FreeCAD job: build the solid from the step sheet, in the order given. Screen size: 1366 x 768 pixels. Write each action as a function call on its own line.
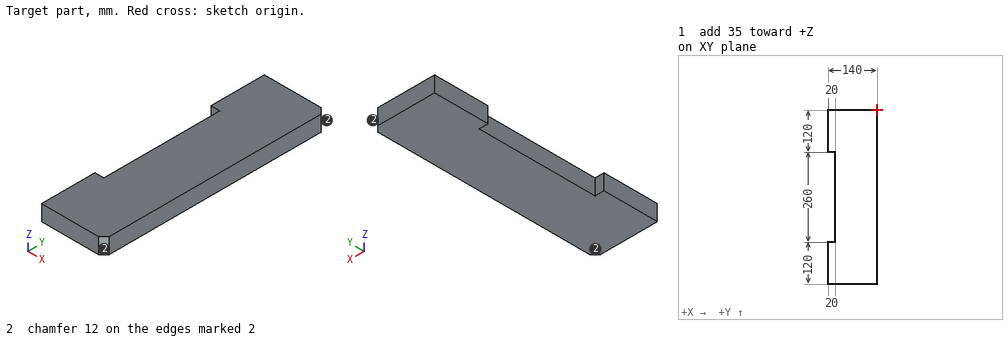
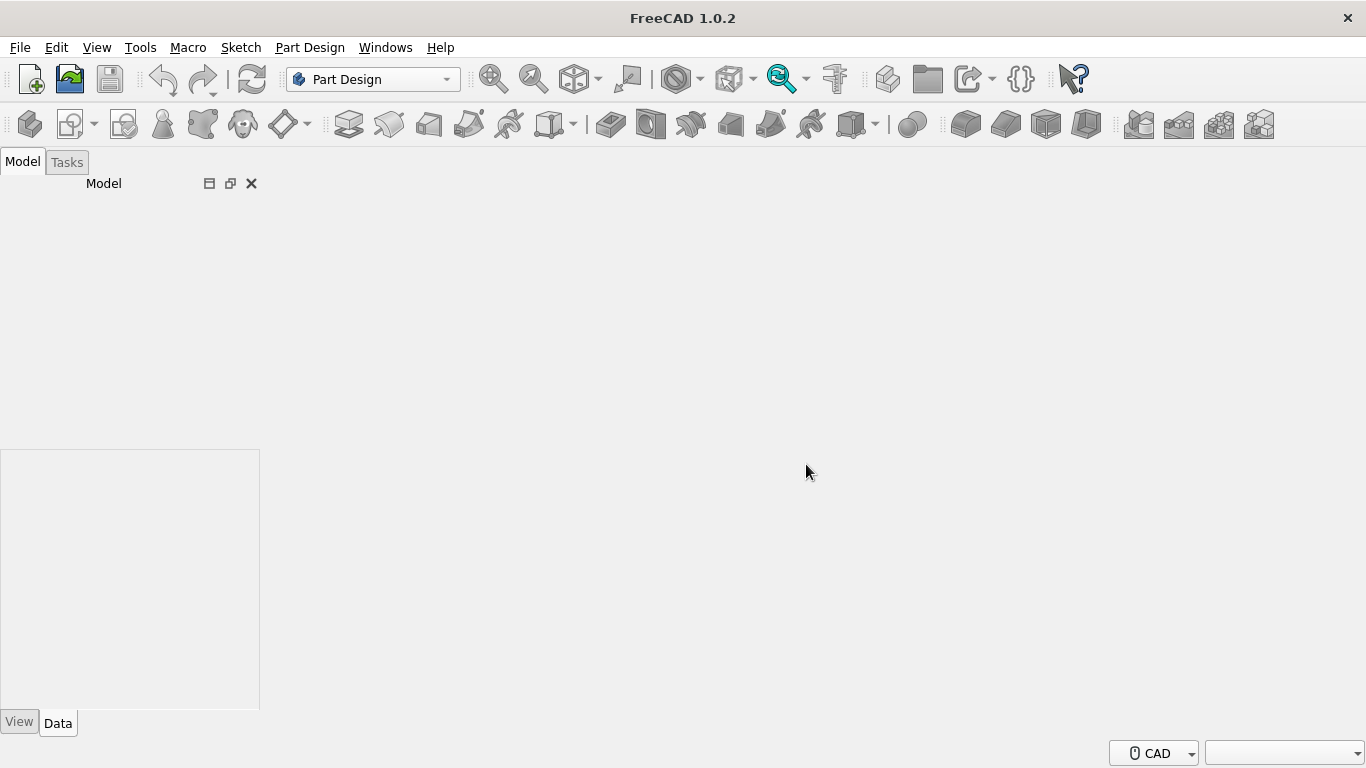
key(ctrl+n)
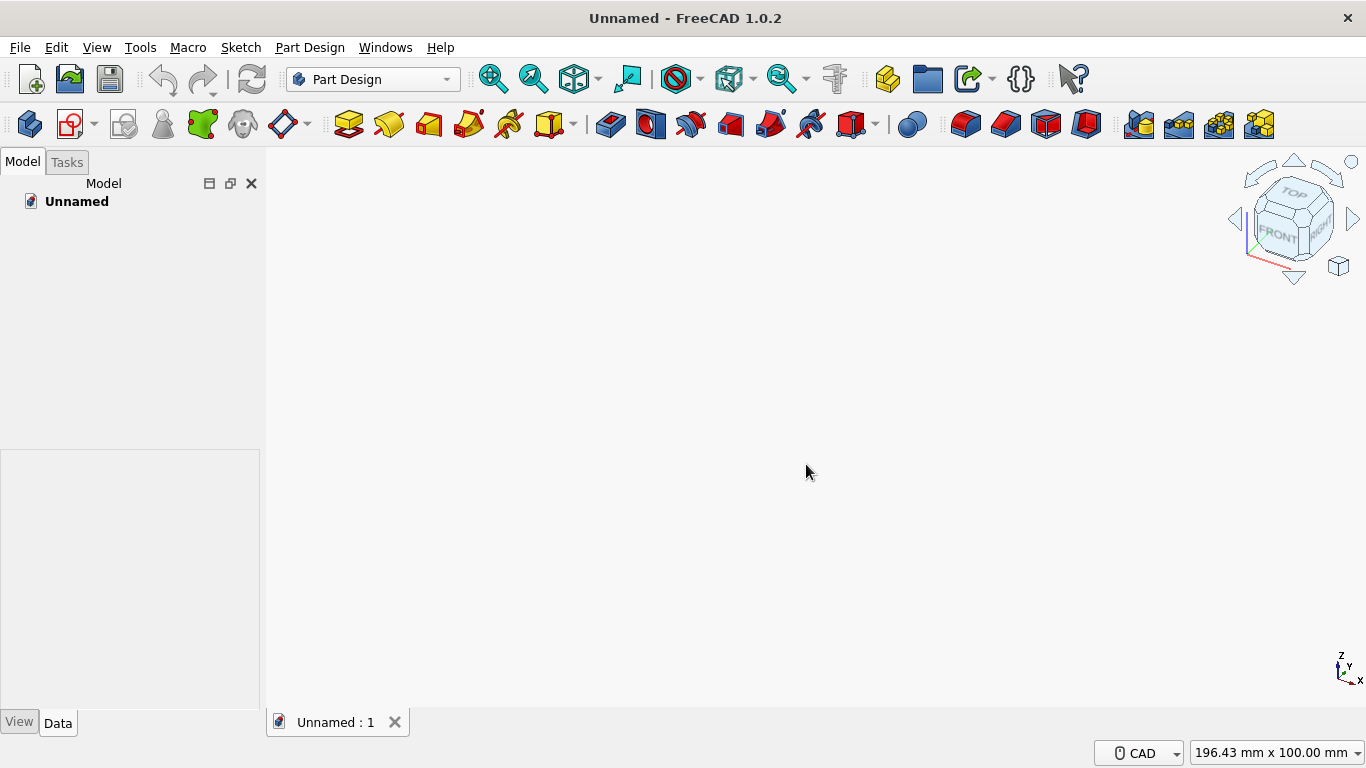
click(70, 124)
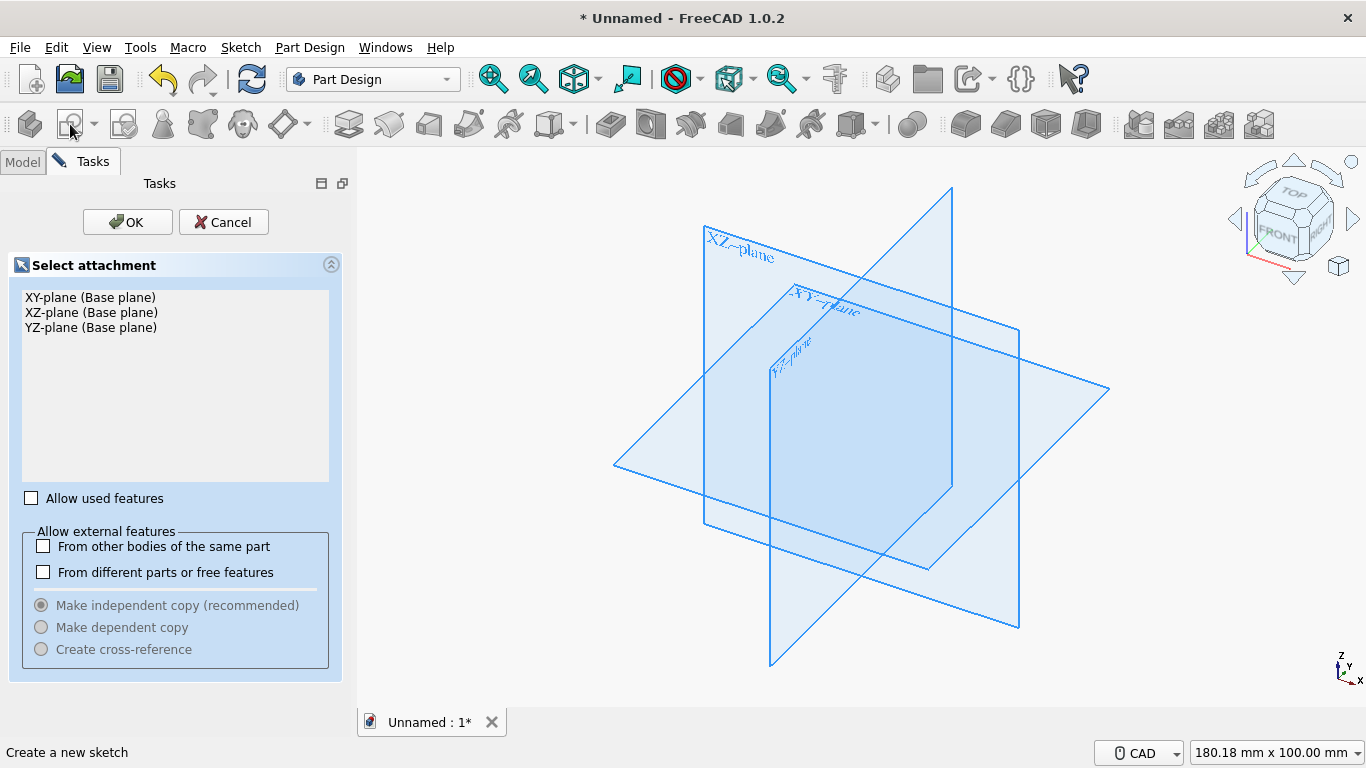
click(82, 298)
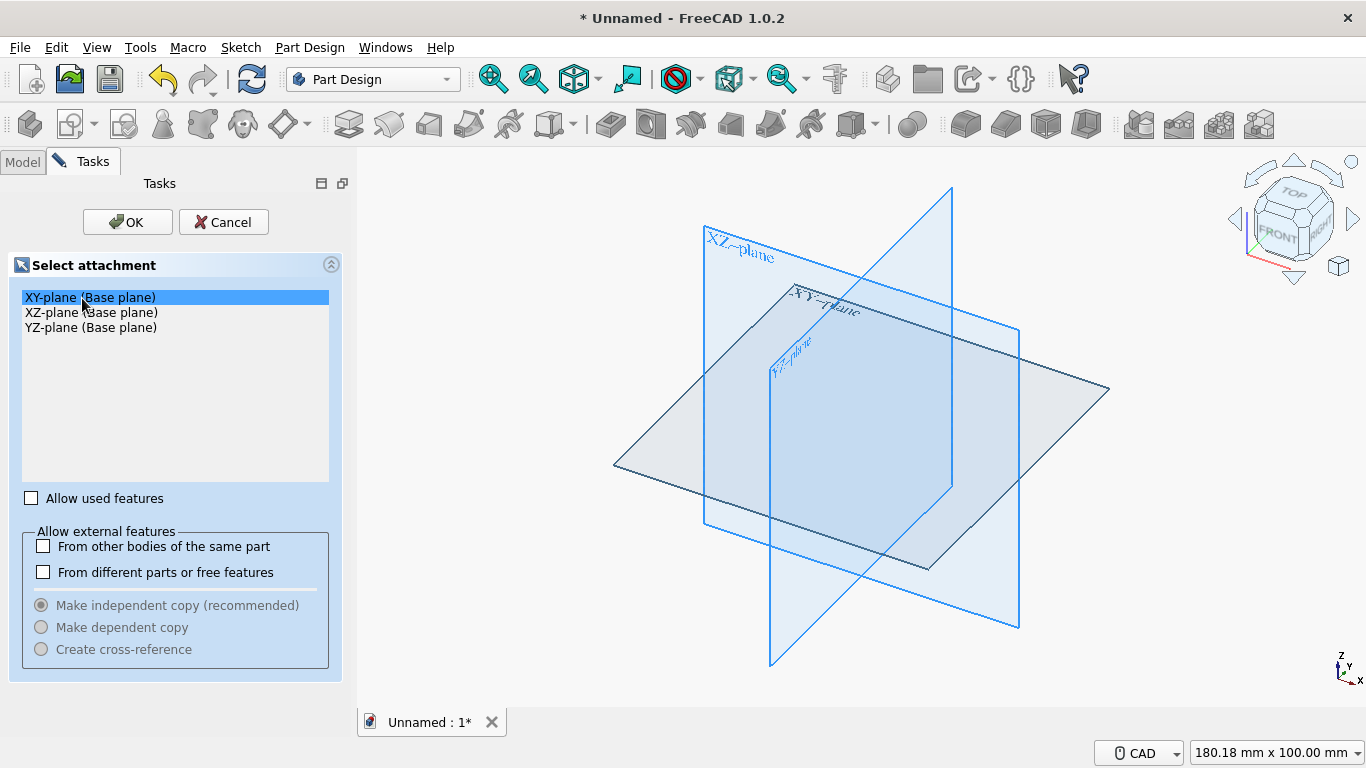
click(128, 222)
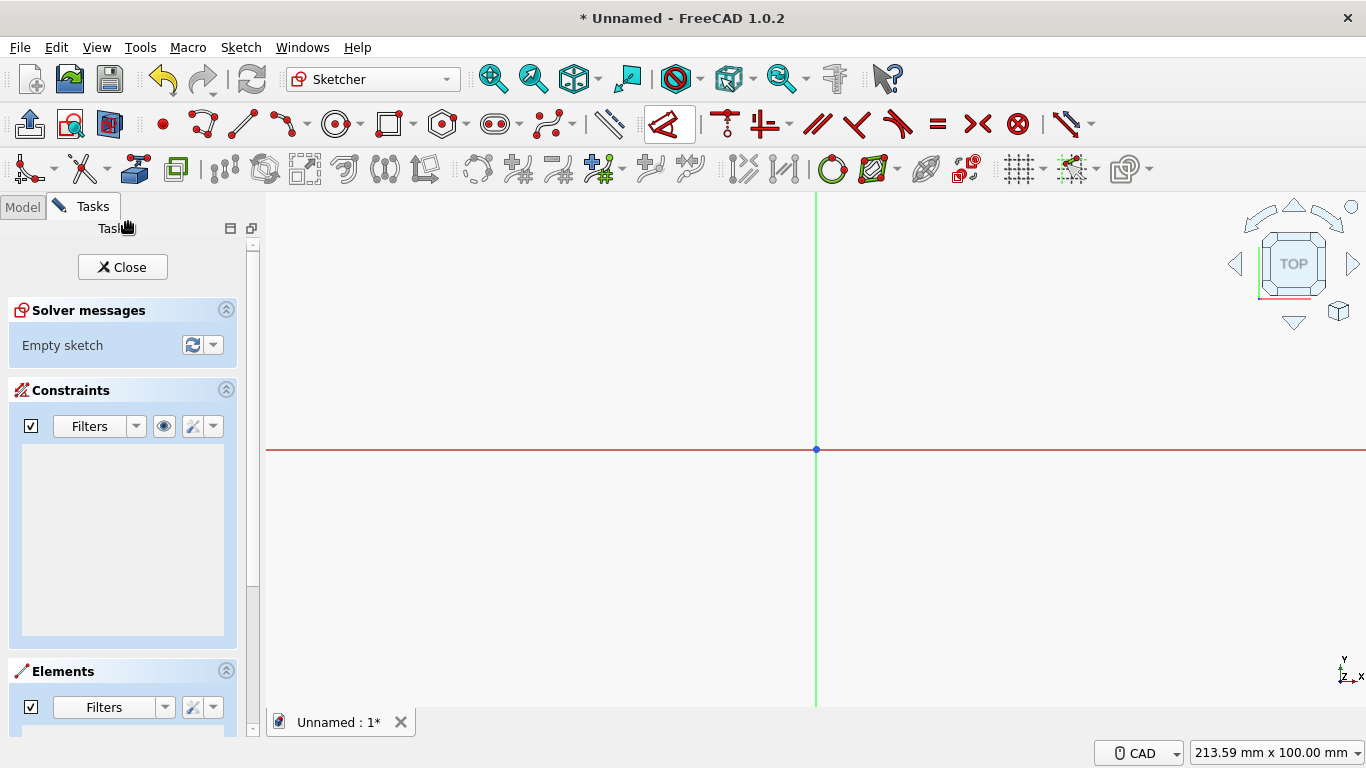
scroll(793, 248, down, 10)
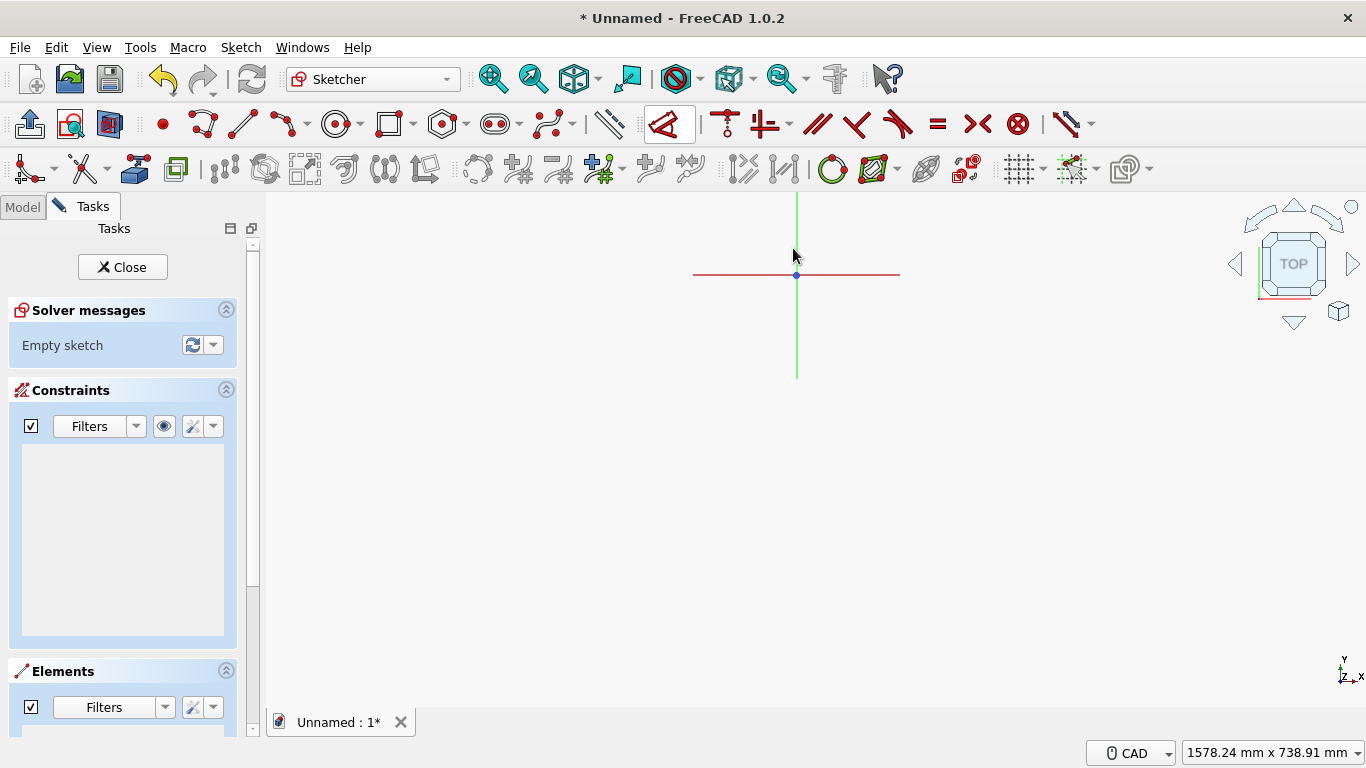
key(g)
key(m)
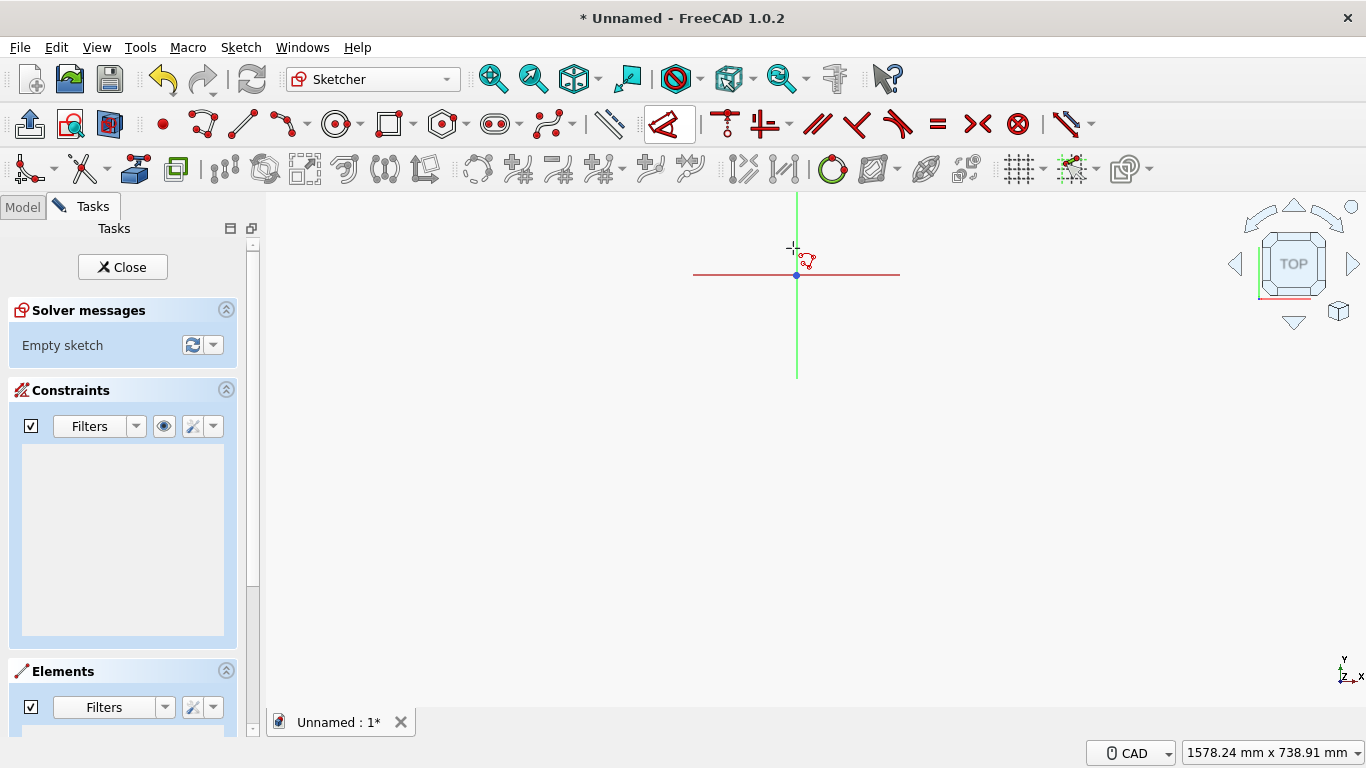
click(797, 275)
click(699, 284)
click(699, 359)
click(713, 359)
click(713, 540)
click(699, 540)
click(699, 624)
click(788, 624)
click(797, 275)
key(Escape)
key(Escape)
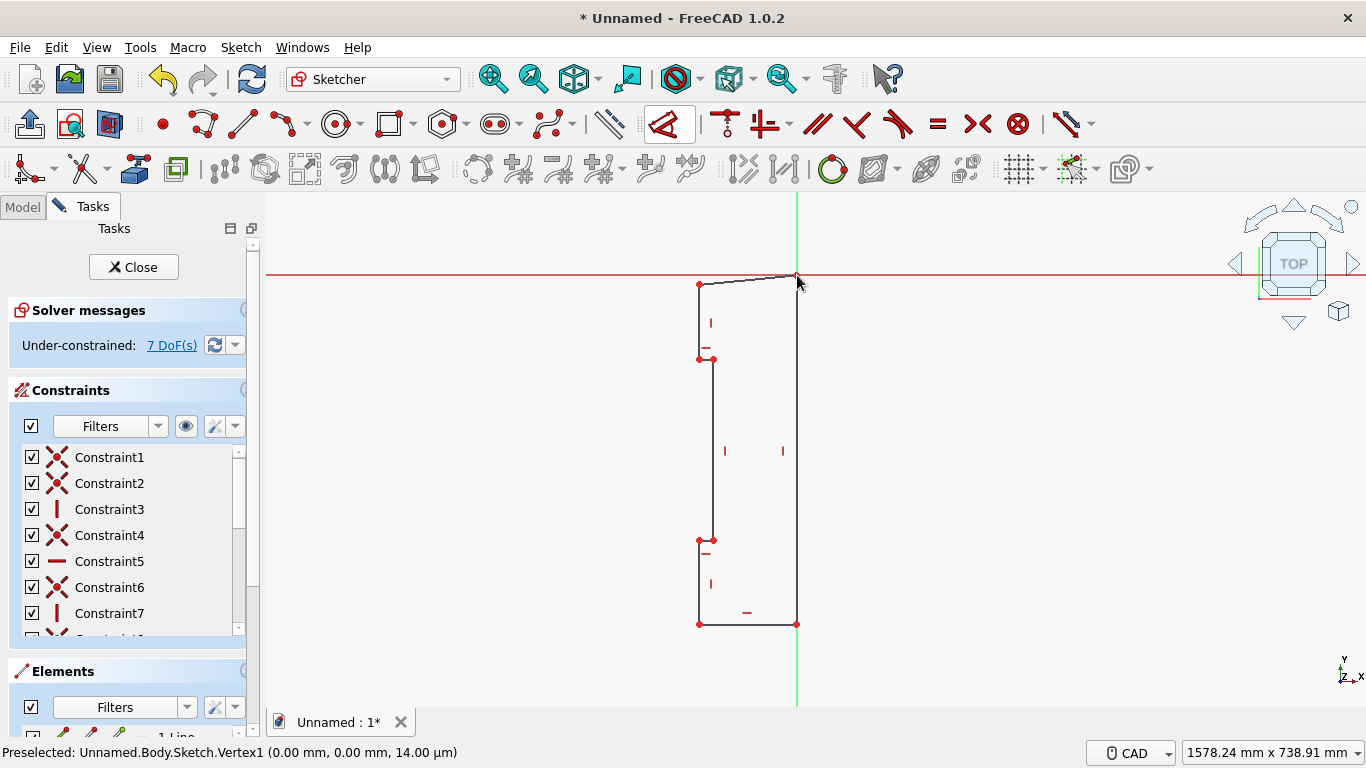
click(767, 278)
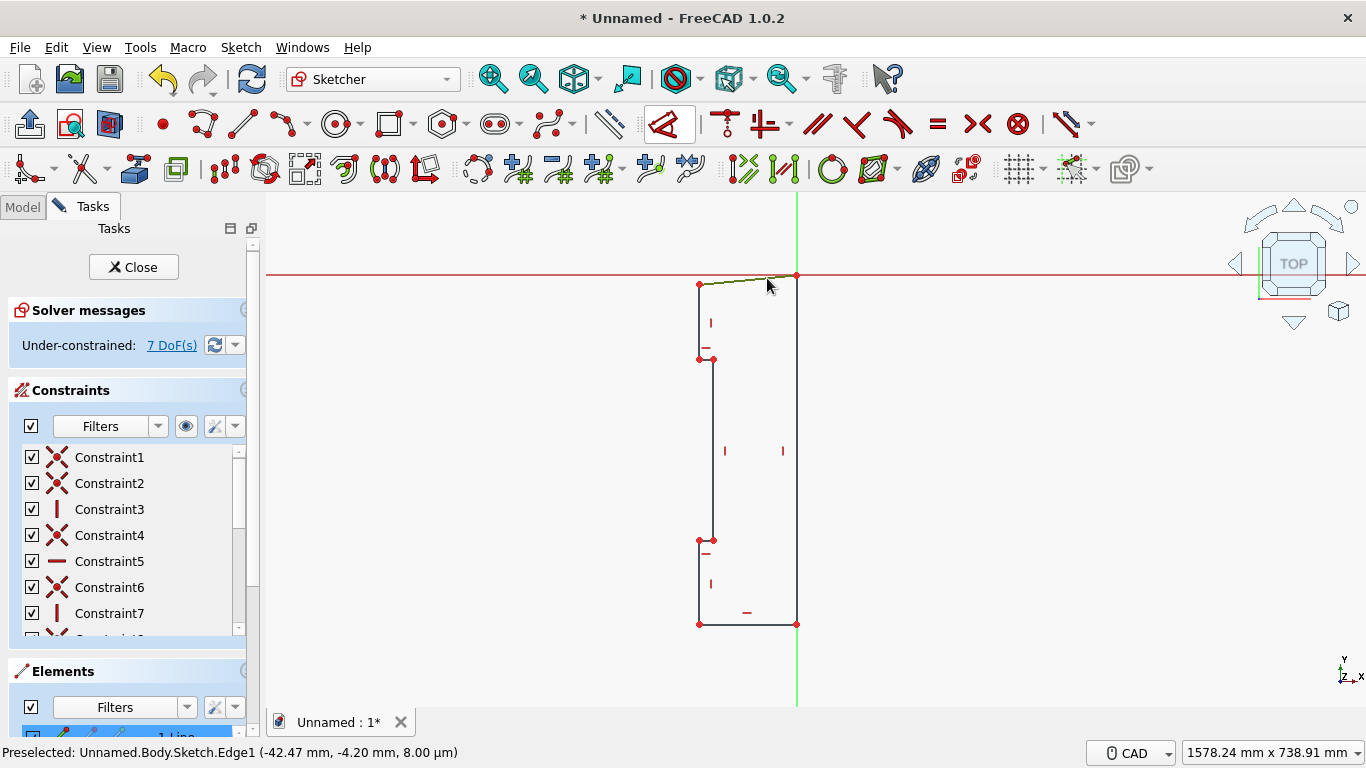
key(h)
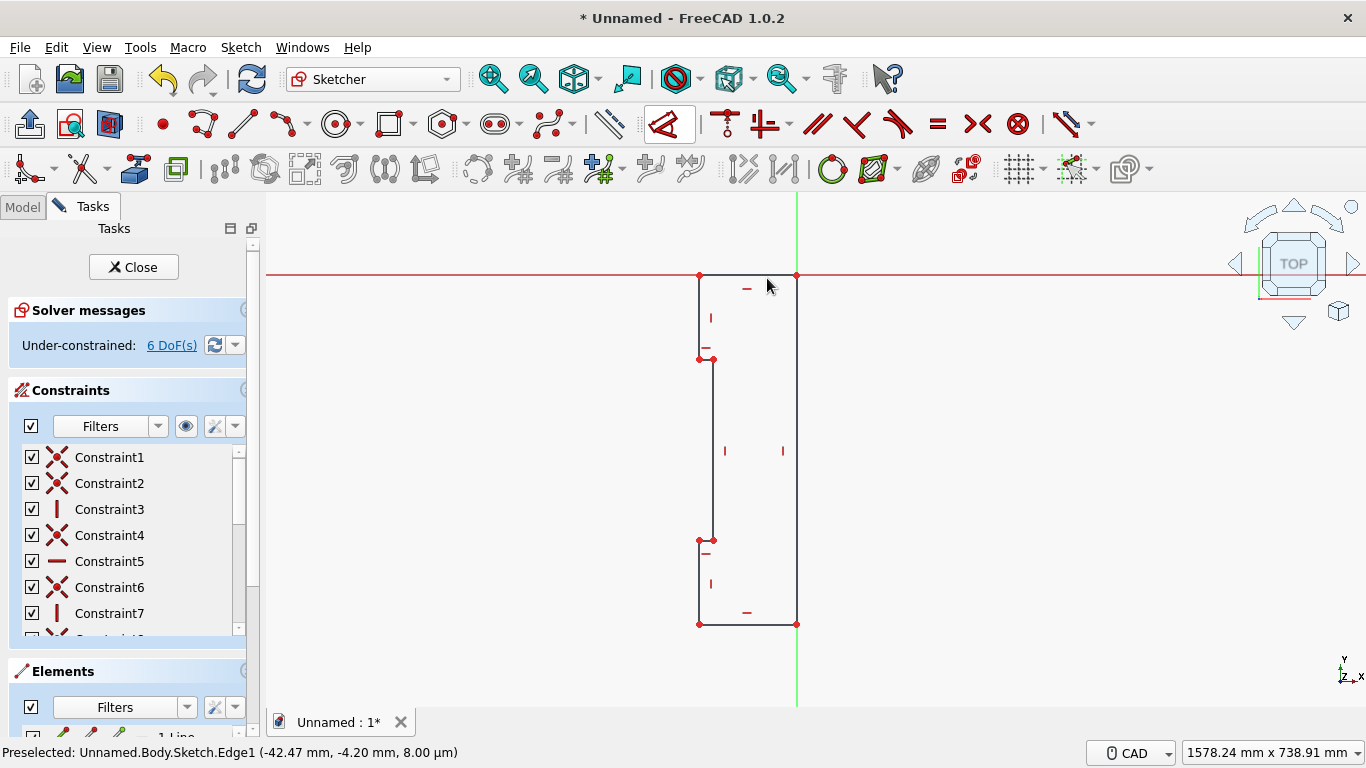
click(664, 124)